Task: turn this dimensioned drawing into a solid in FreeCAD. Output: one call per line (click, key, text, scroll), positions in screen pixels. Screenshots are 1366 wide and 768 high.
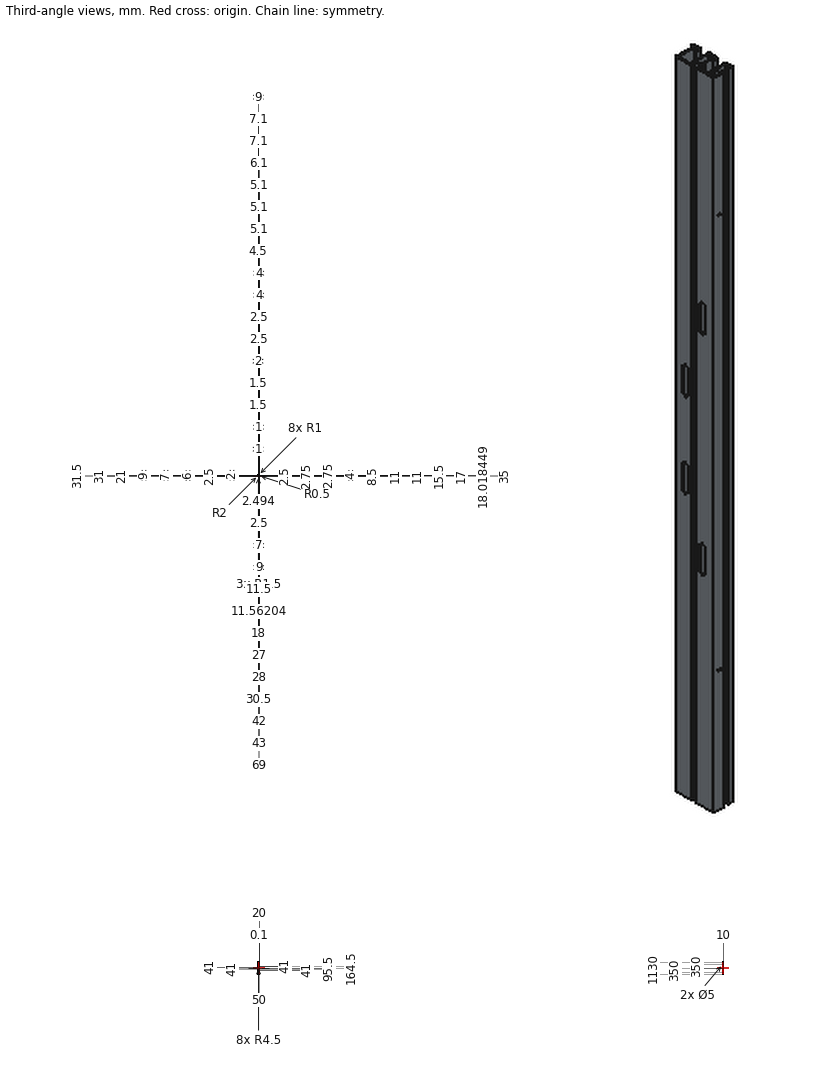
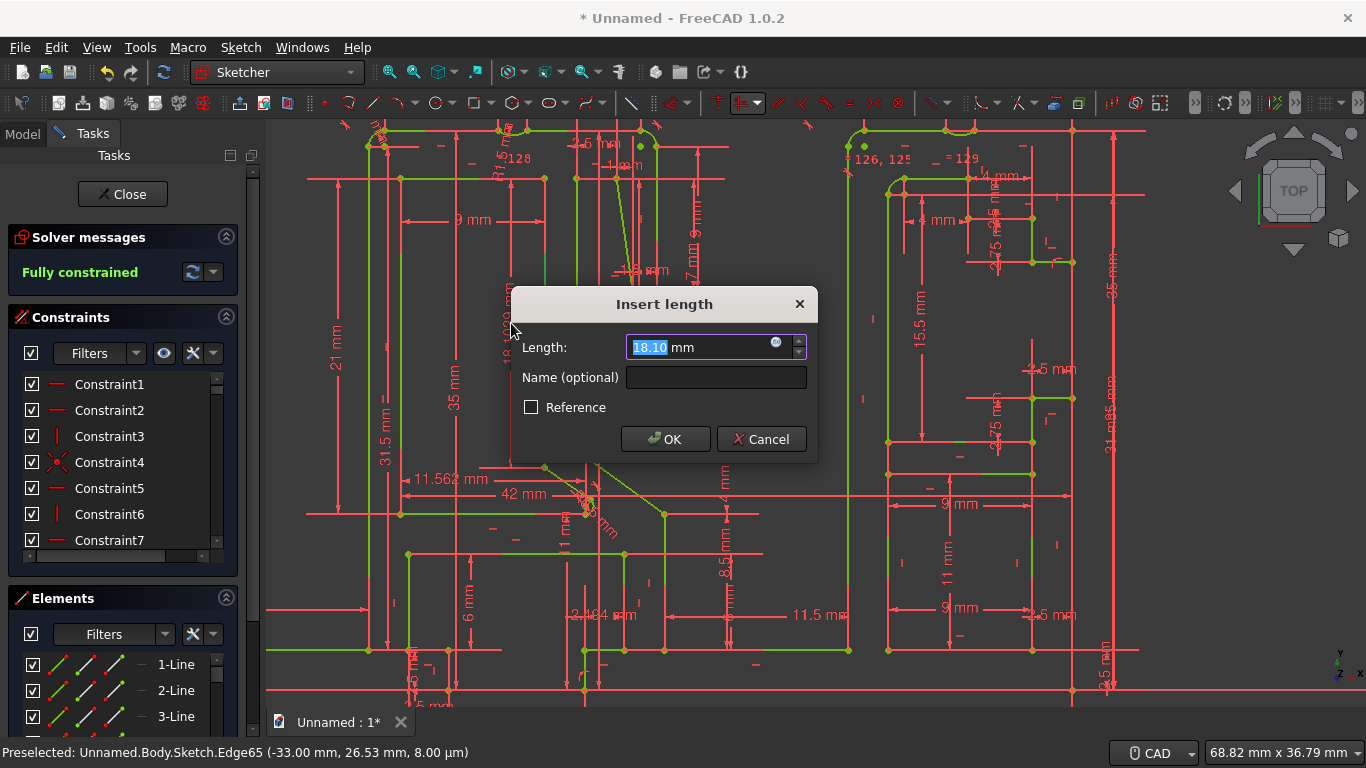
text(18.018449)
key(Return)
key(Escape)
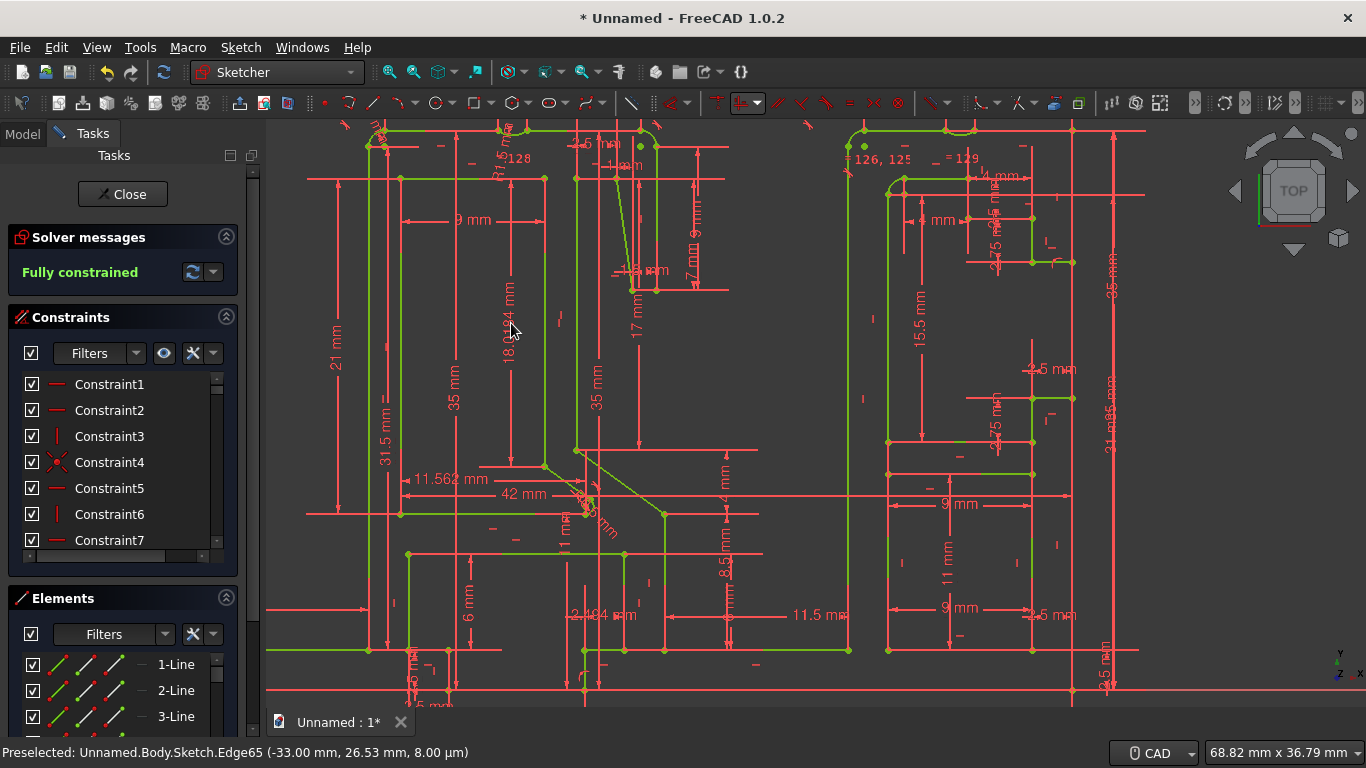
click(123, 194)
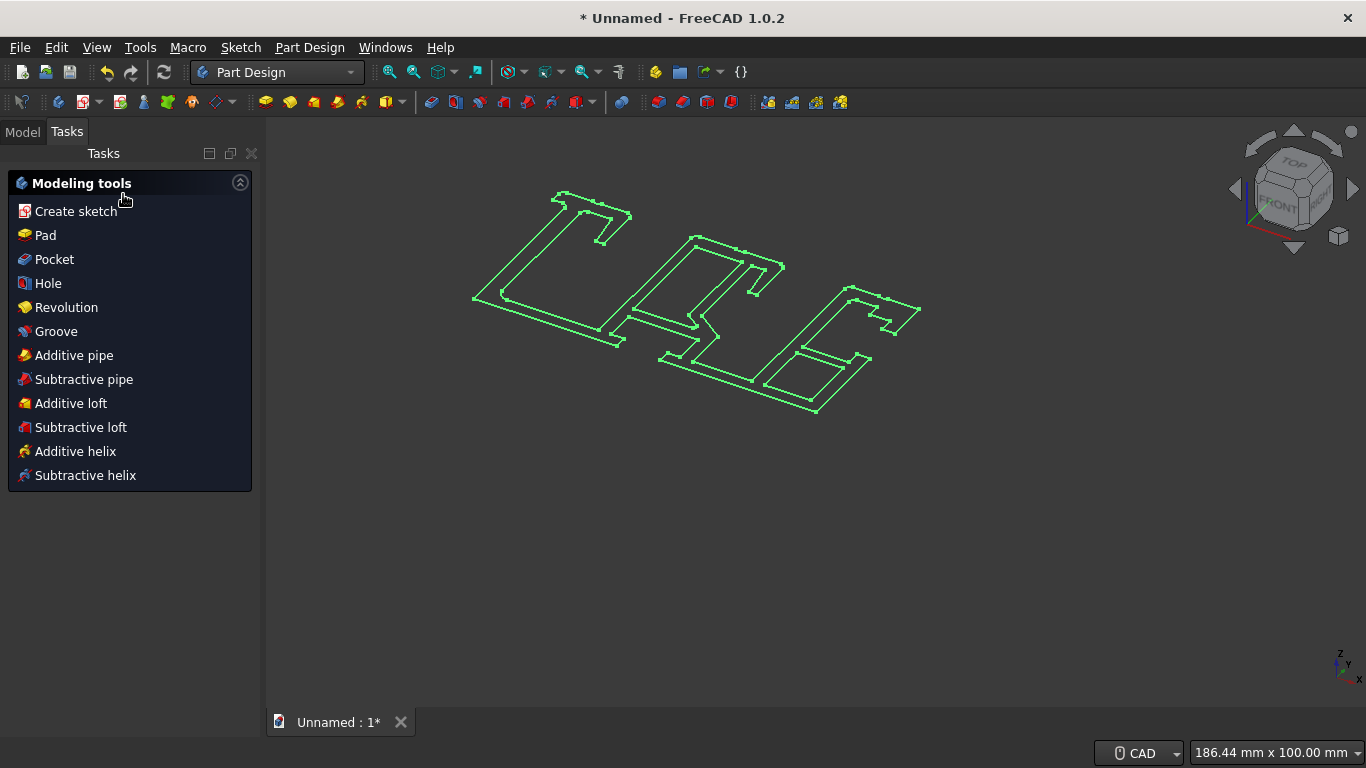
click(266, 102)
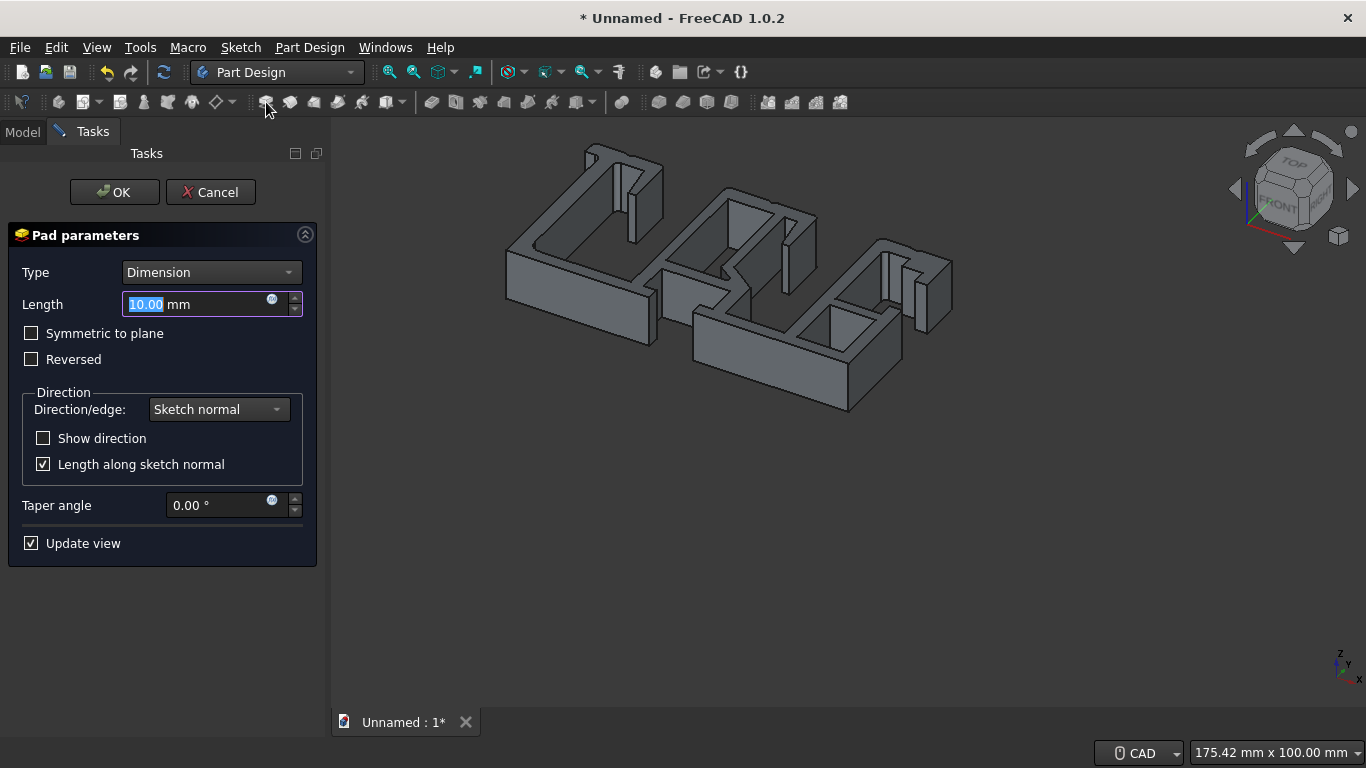
text(1130)
key(Tab)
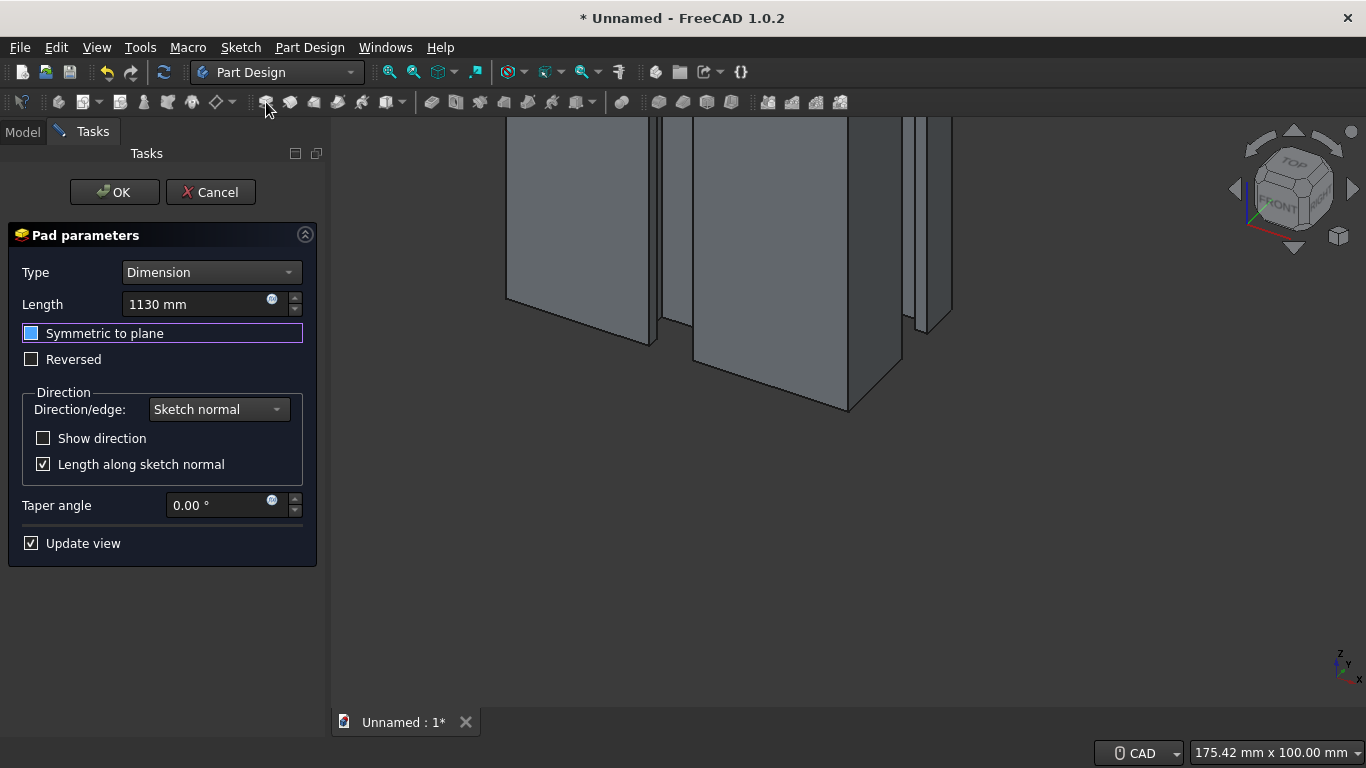
click(30, 333)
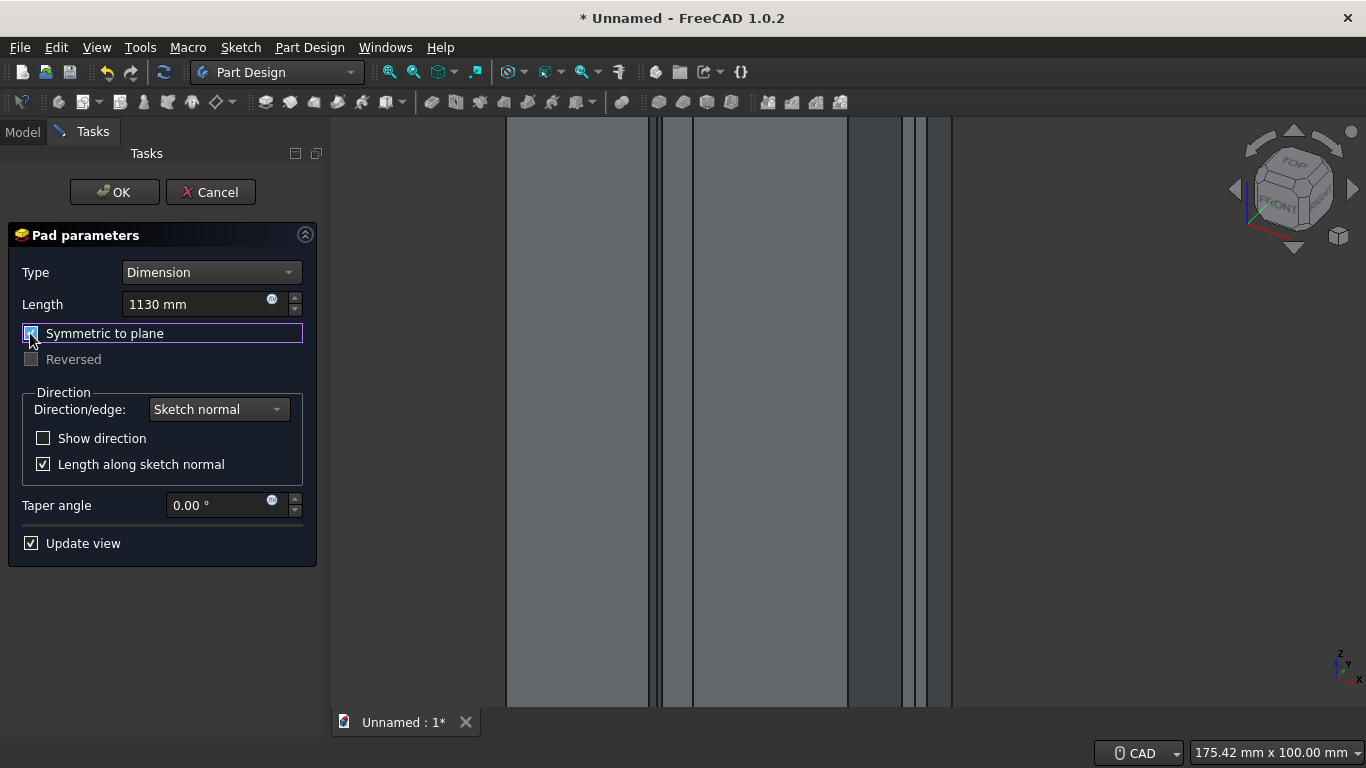
click(115, 192)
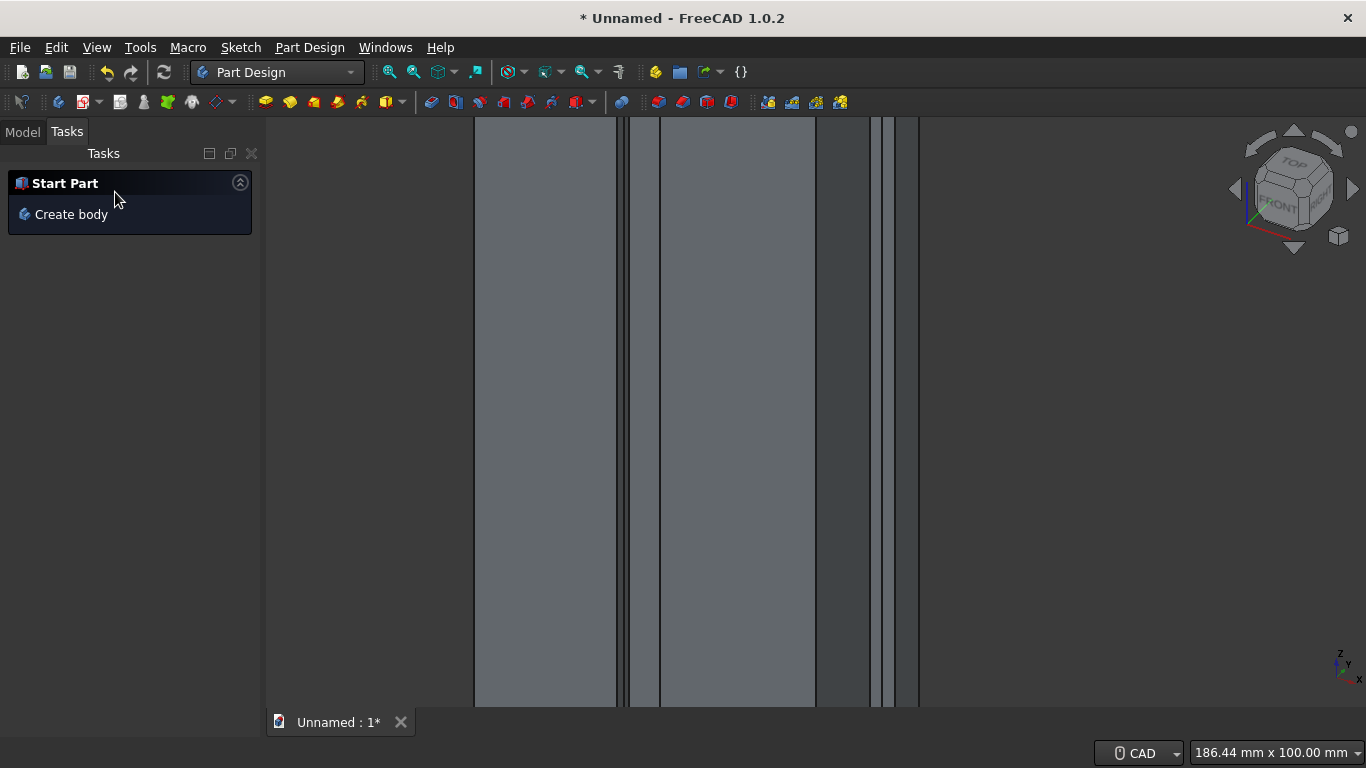
key(v)
key(f)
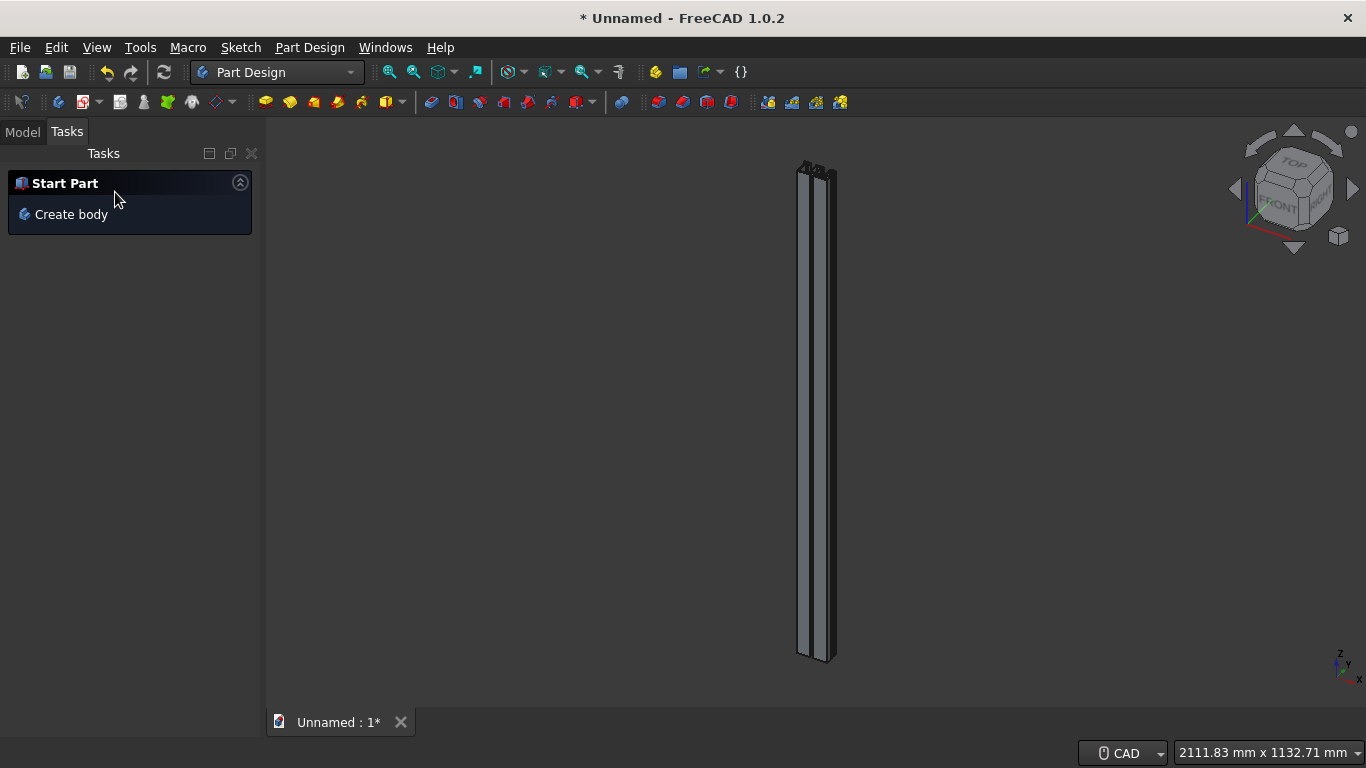
key(4)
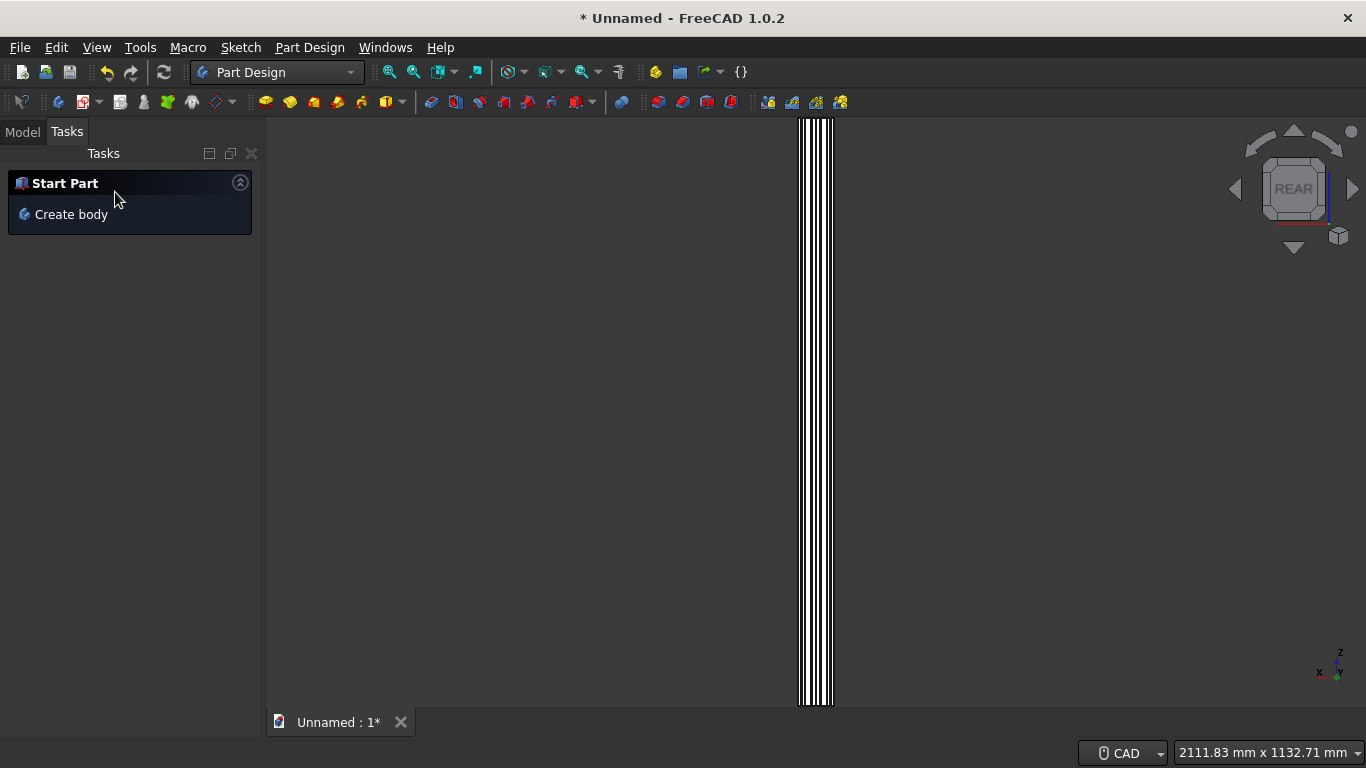
scroll(825, 159, up, 5)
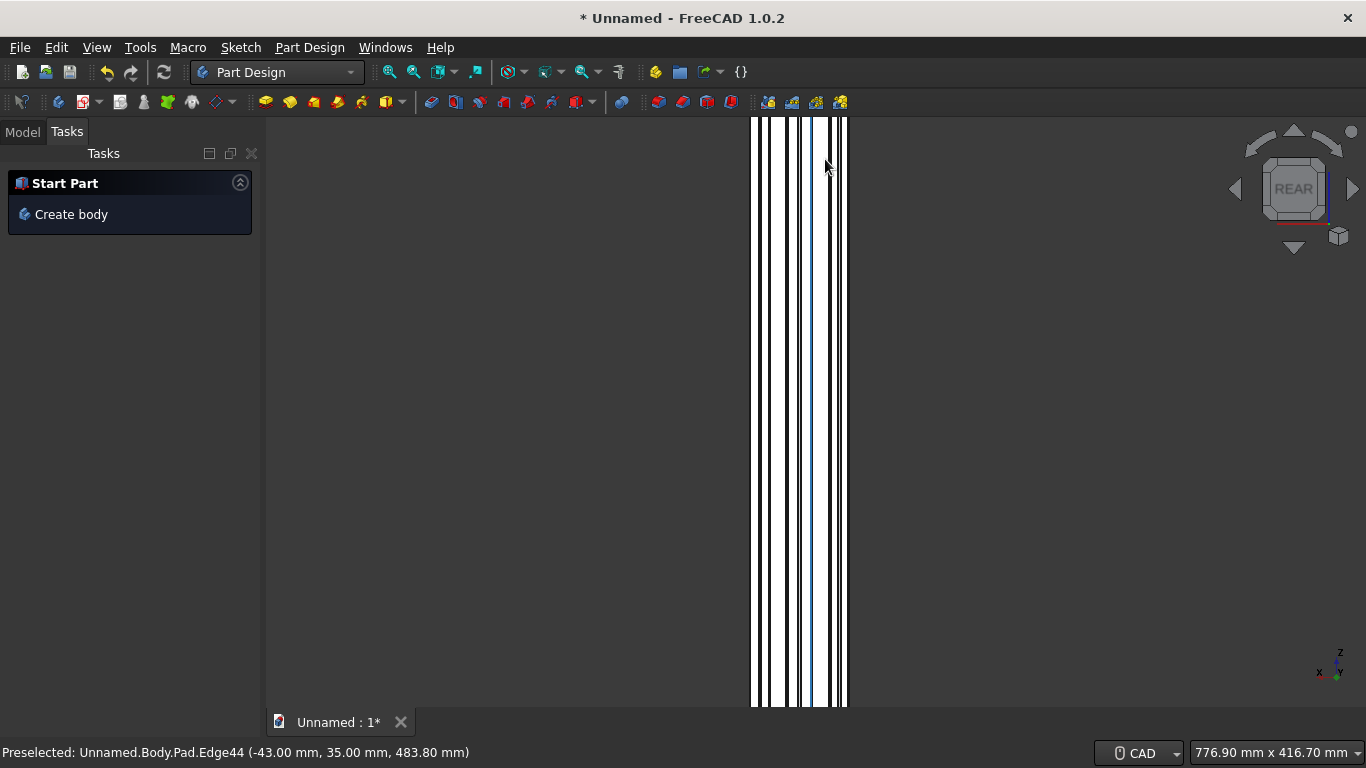
click(390, 72)